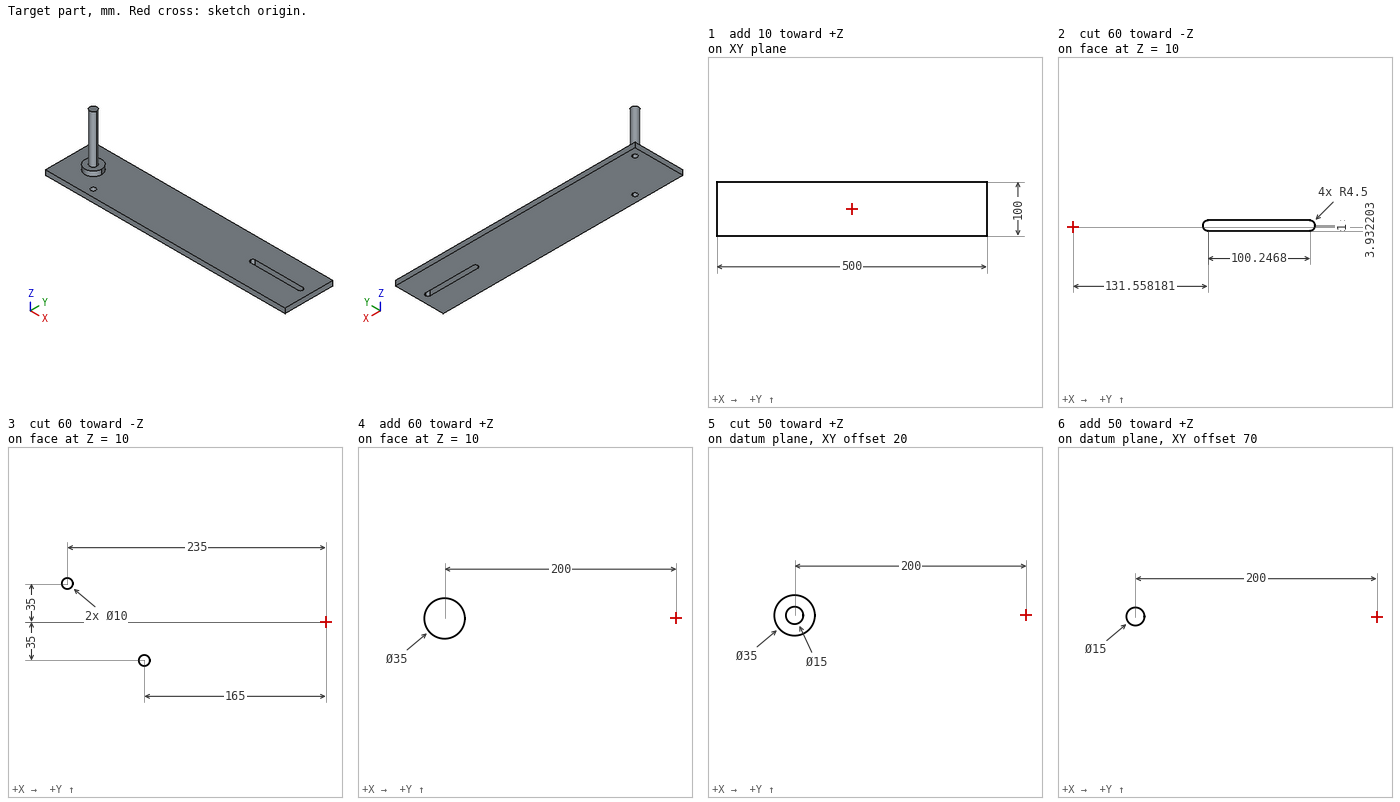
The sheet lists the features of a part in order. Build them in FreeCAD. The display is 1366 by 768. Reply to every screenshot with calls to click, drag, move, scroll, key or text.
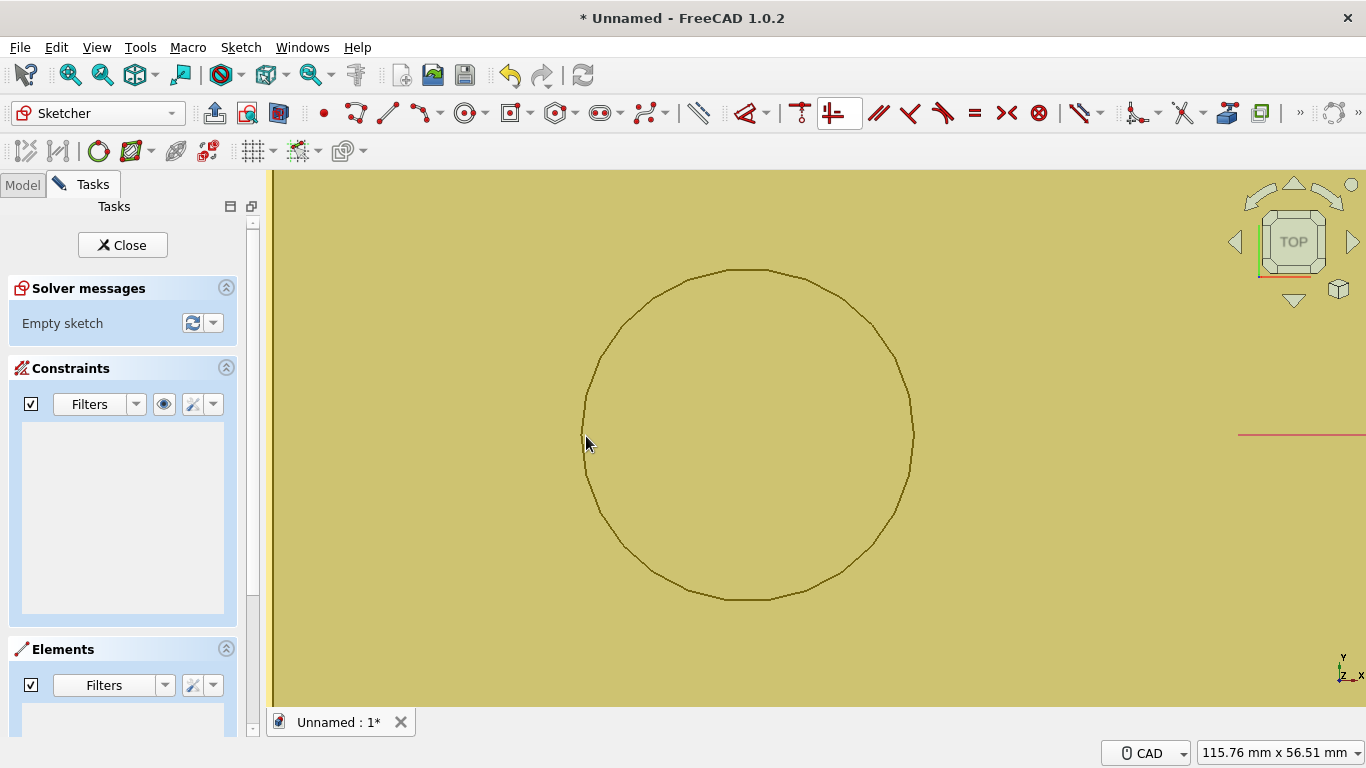
key(g)
key(c)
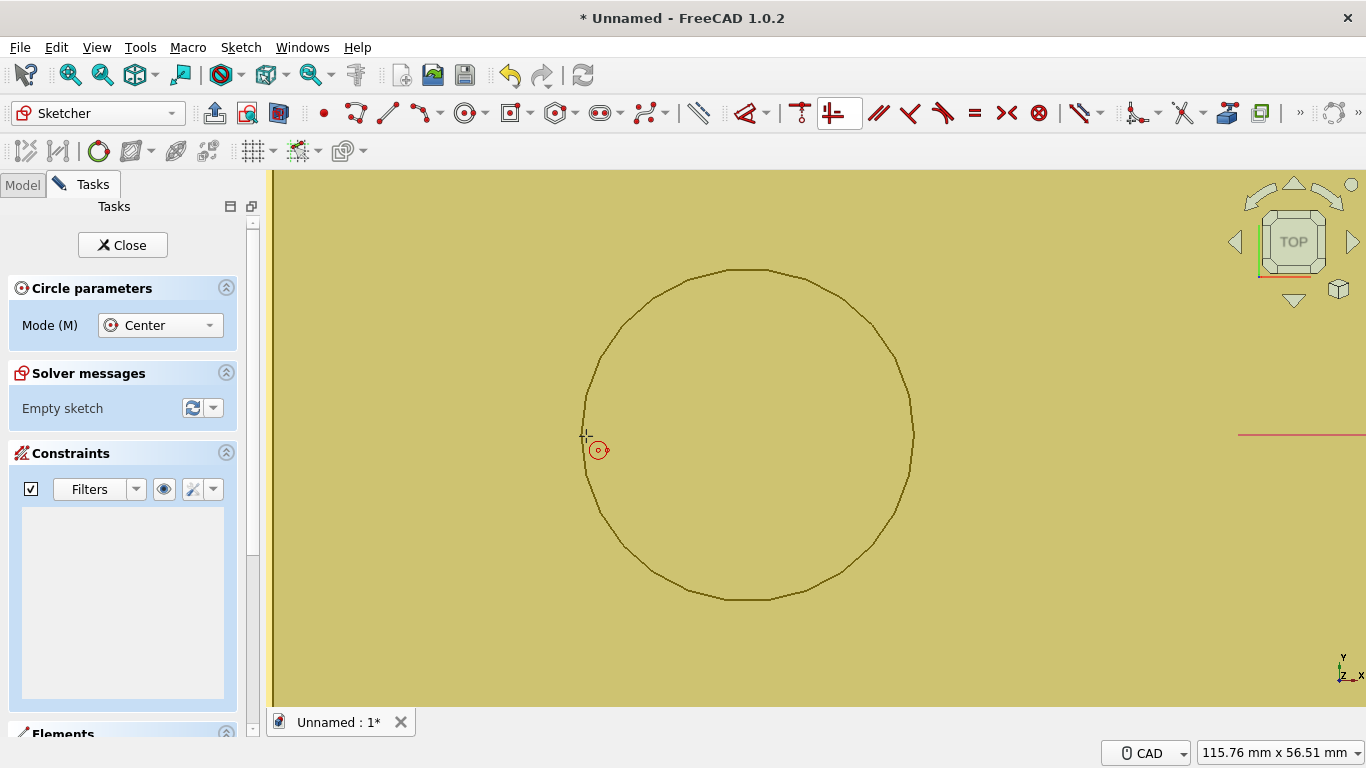
click(748, 435)
move(865, 318)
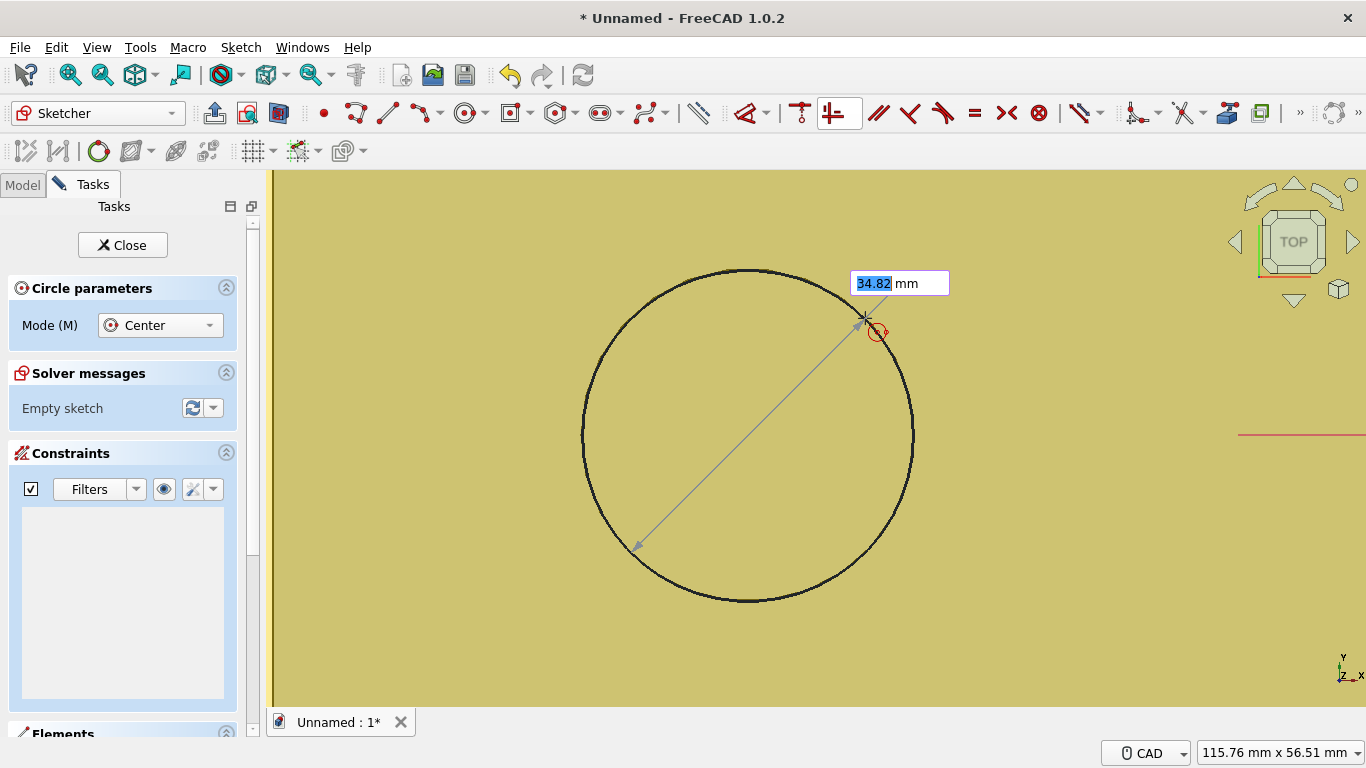
text(35)
key(Return)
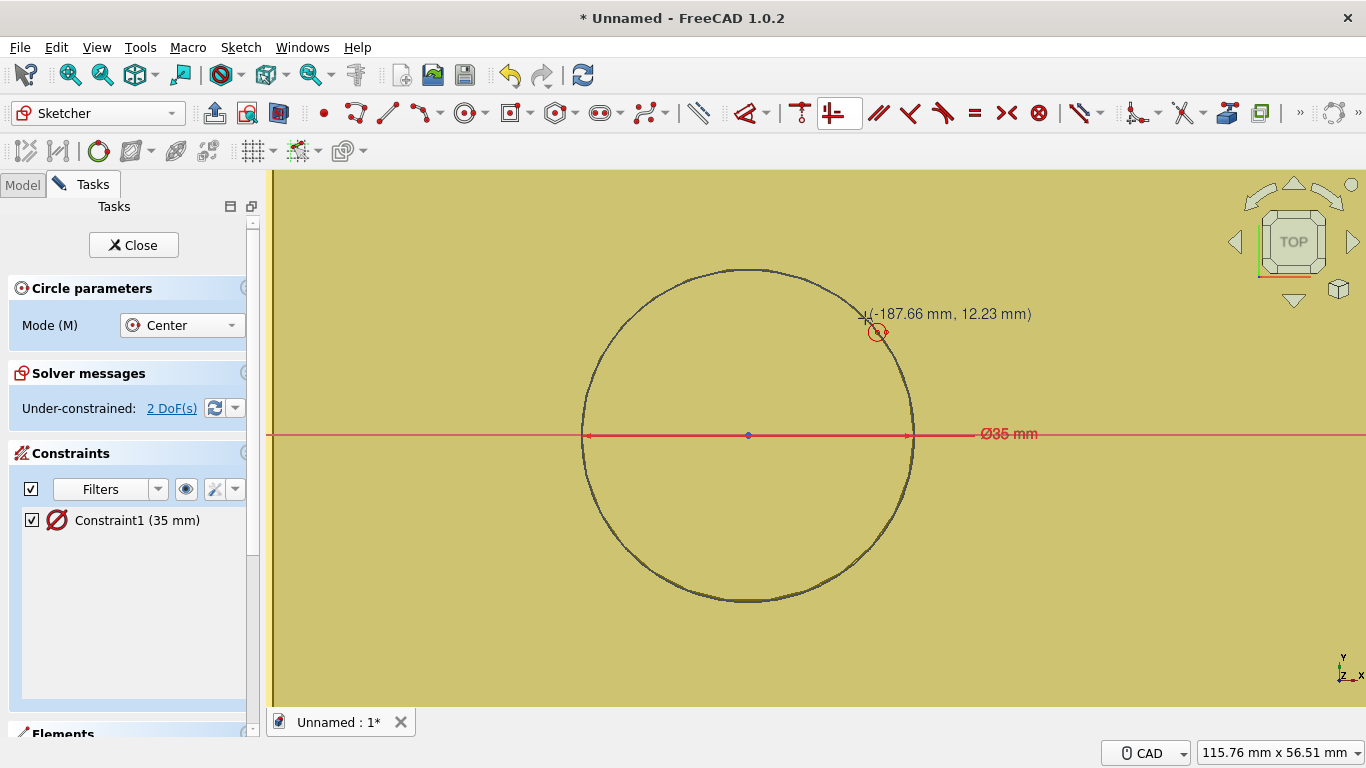
click(748, 436)
move(798, 385)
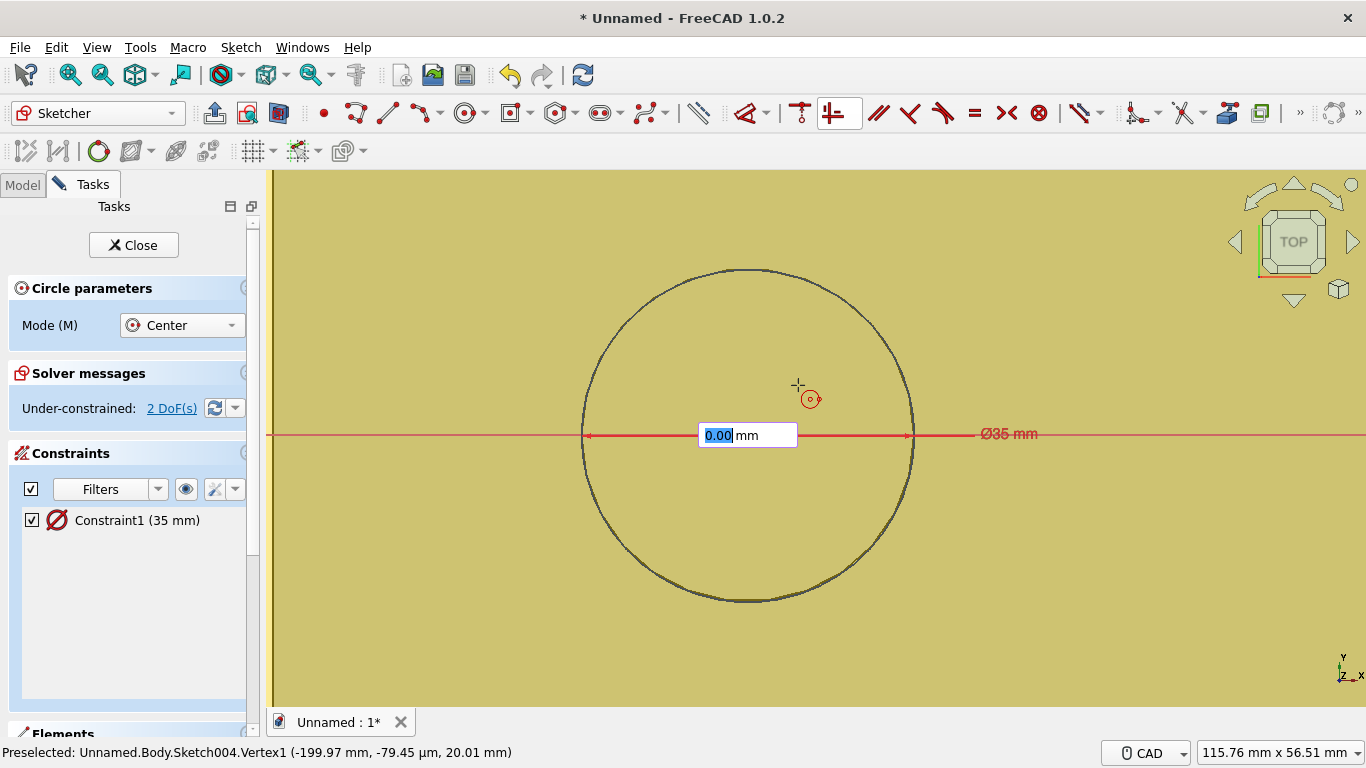
text(15)
key(Return)
key(Escape)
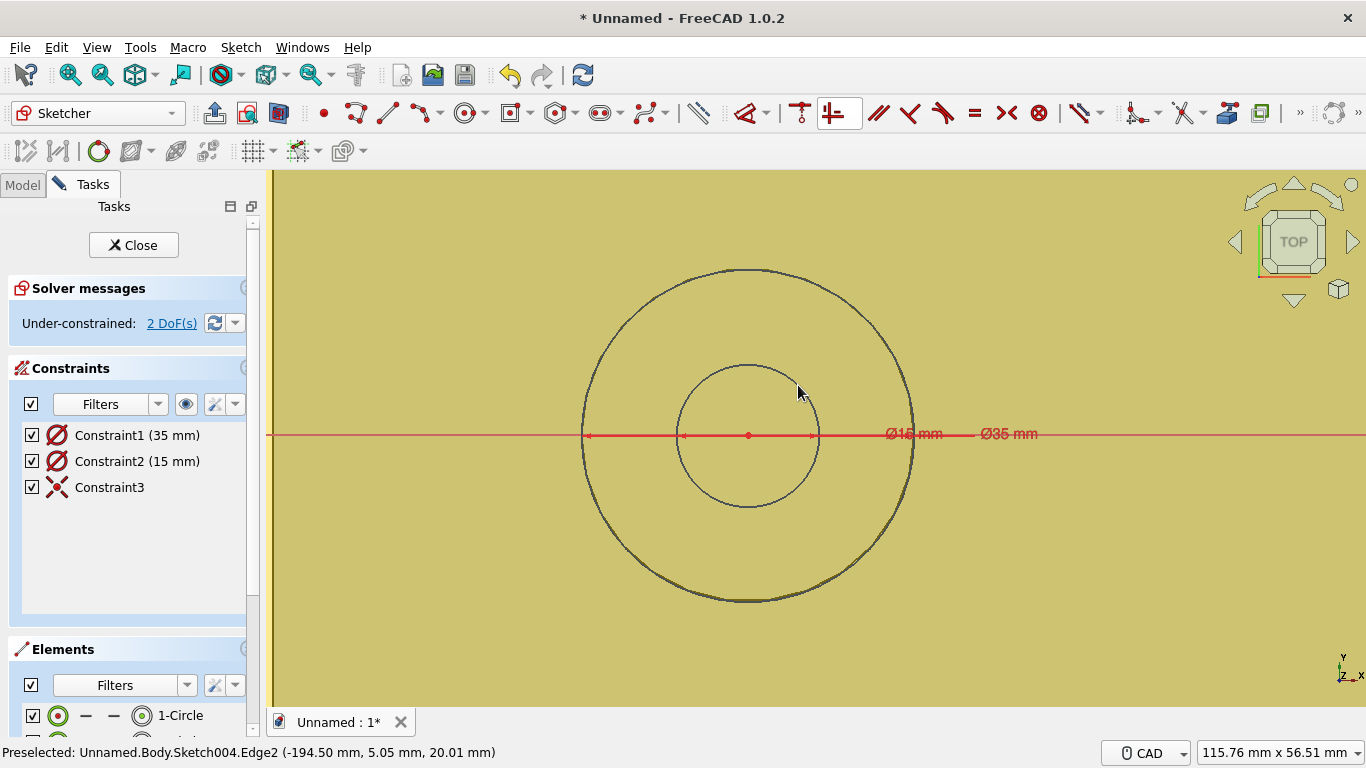
click(748, 436)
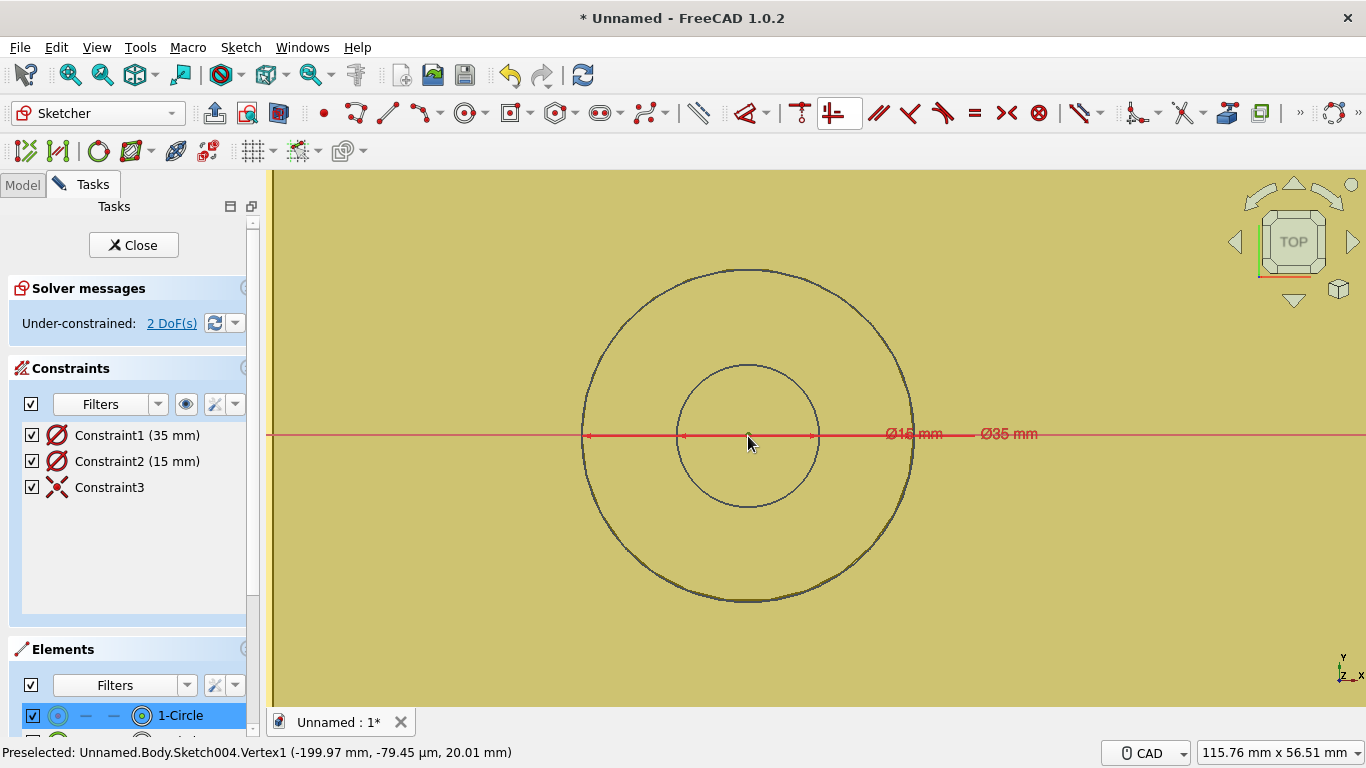
click(359, 435)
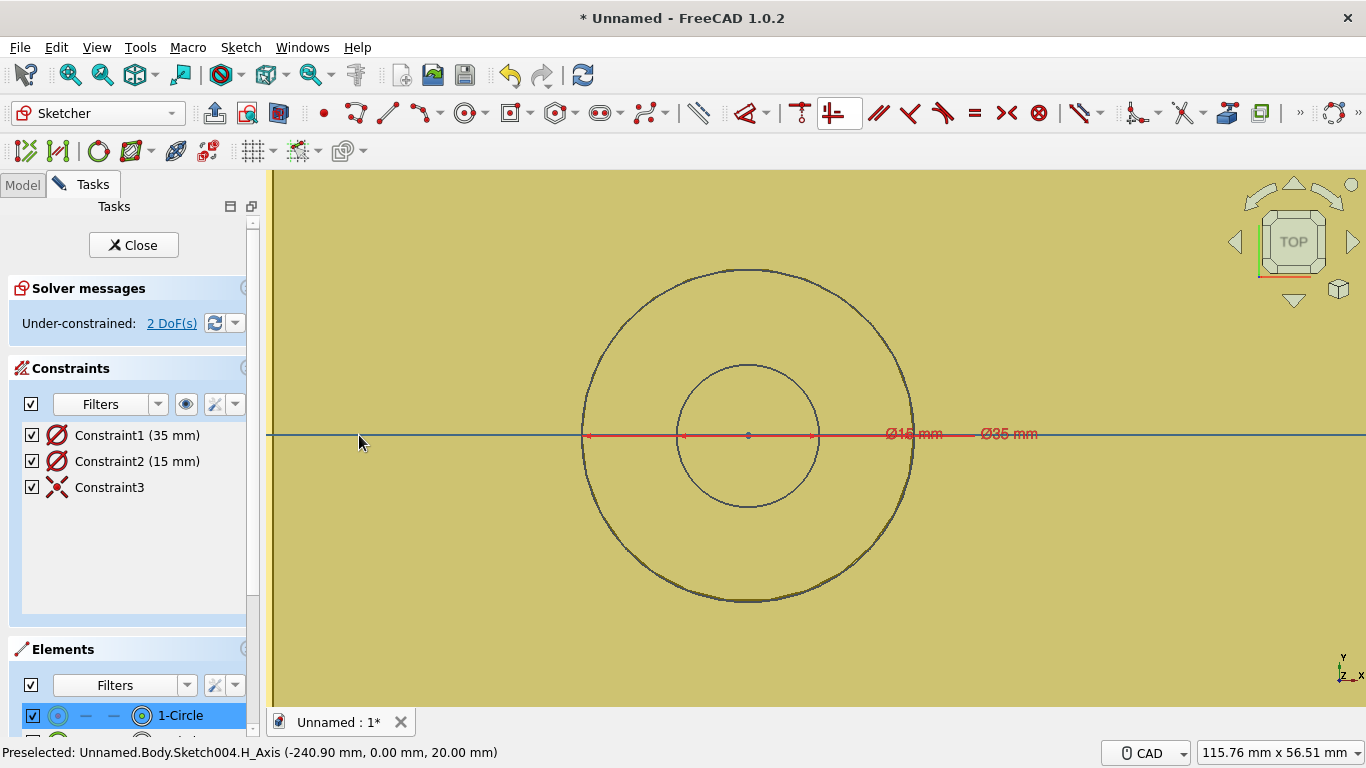
key(c)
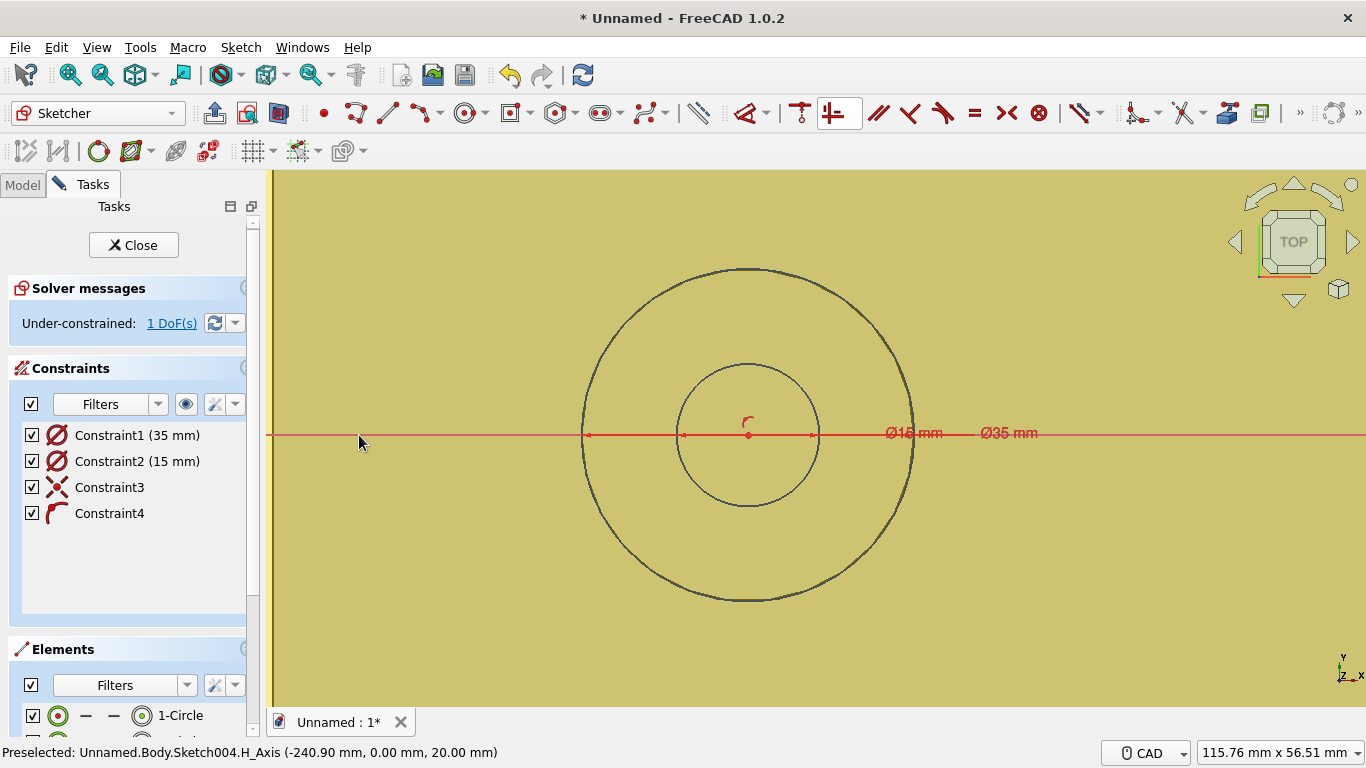
key(d)